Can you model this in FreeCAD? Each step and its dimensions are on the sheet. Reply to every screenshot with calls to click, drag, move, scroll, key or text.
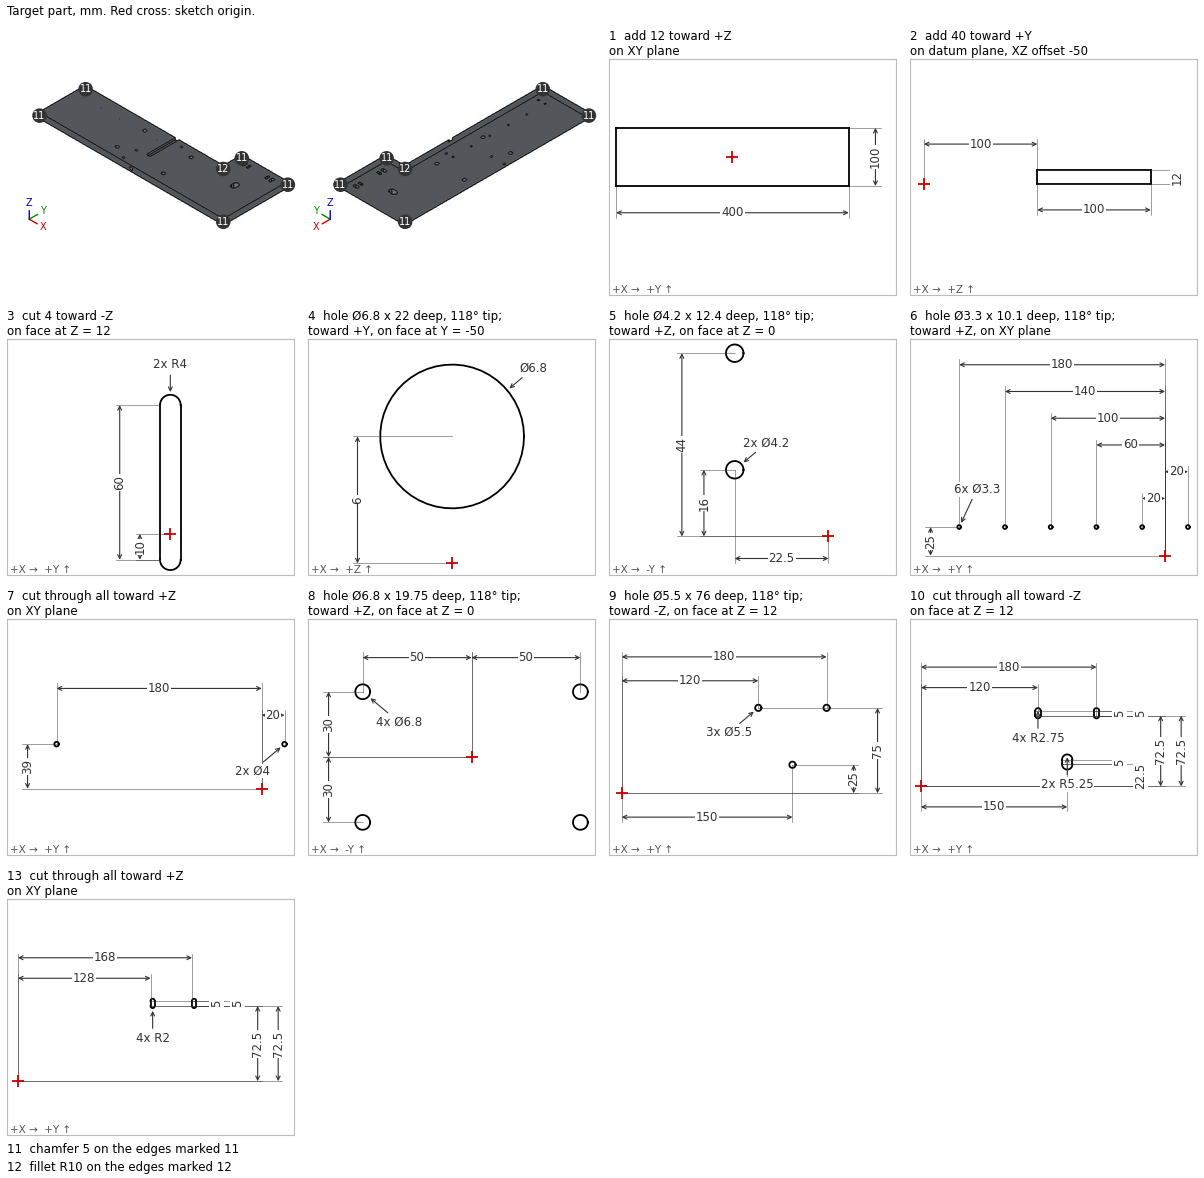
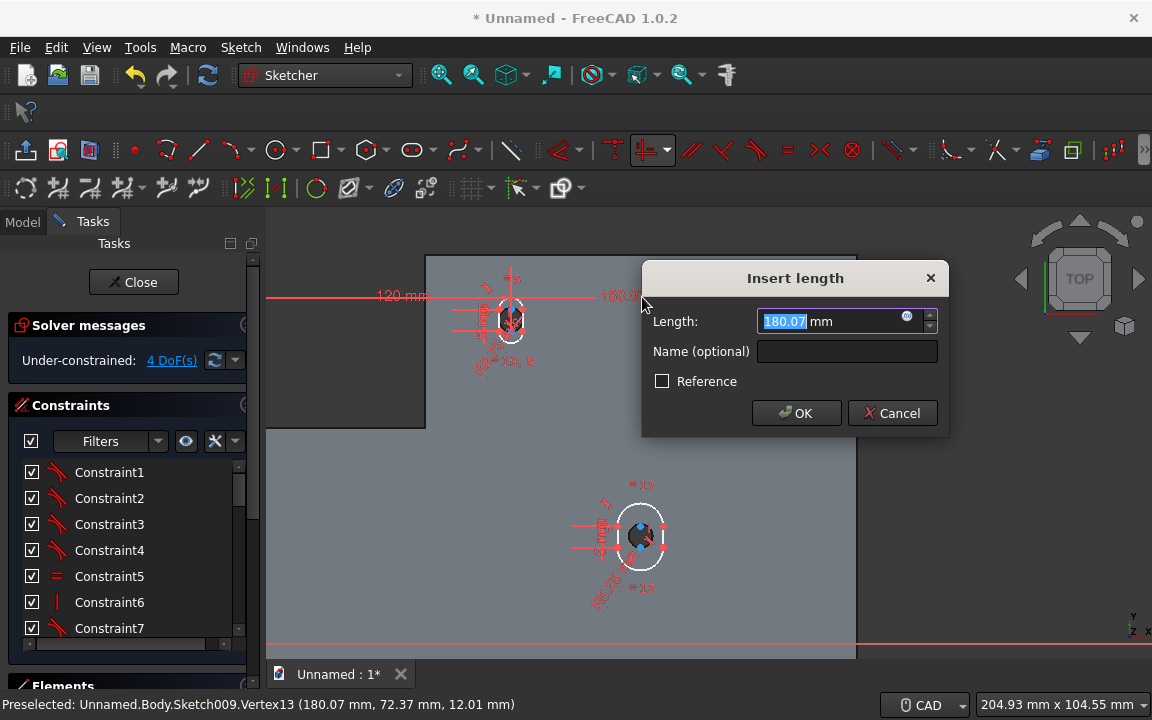
text(180)
key(Return)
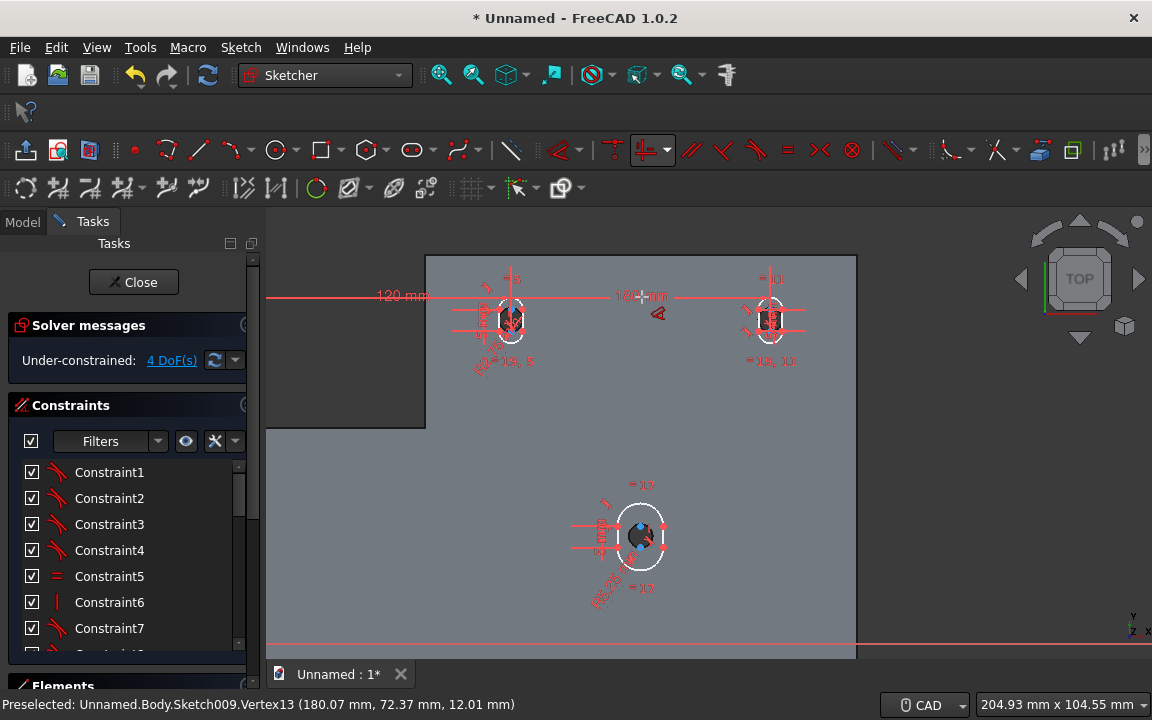
click(640, 548)
click(467, 514)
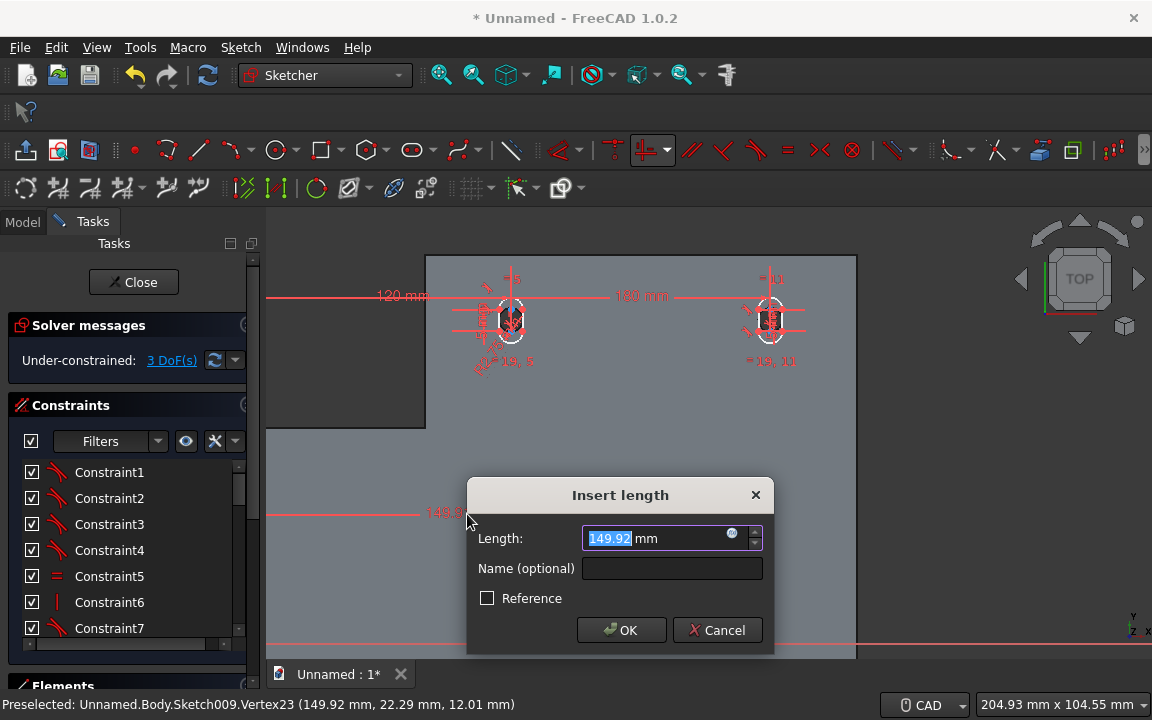
text(150)
key(Return)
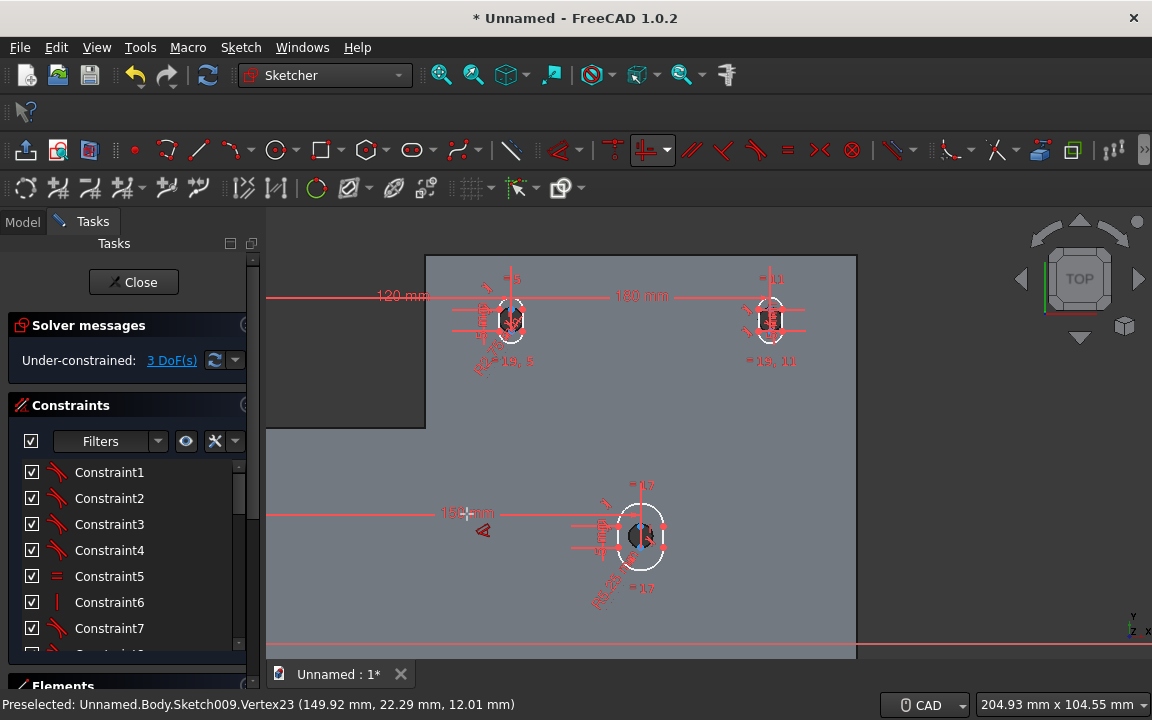
click(499, 331)
click(533, 481)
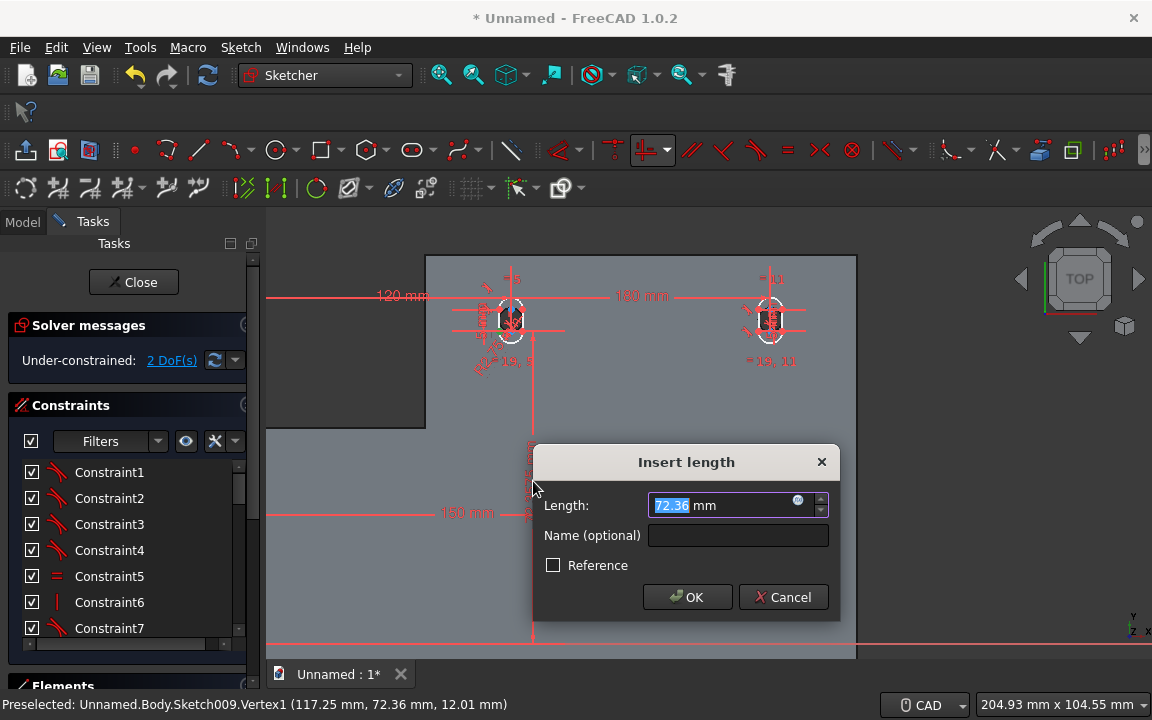
text(72.5)
key(Return)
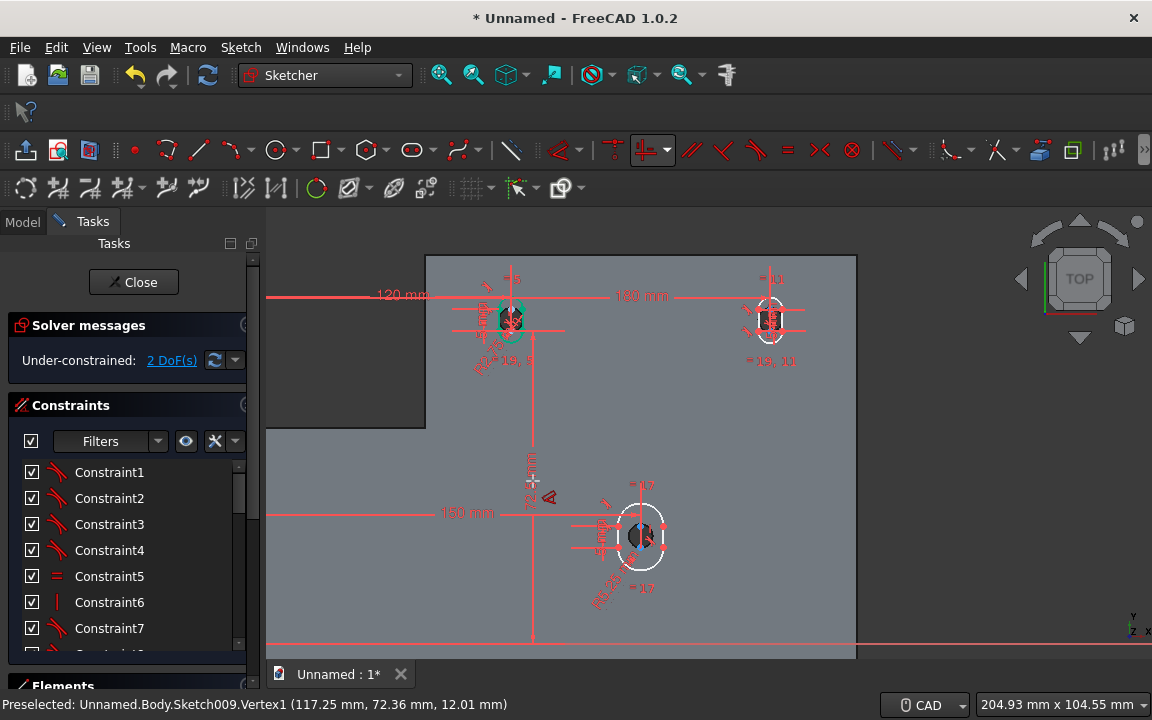
click(759, 331)
click(793, 481)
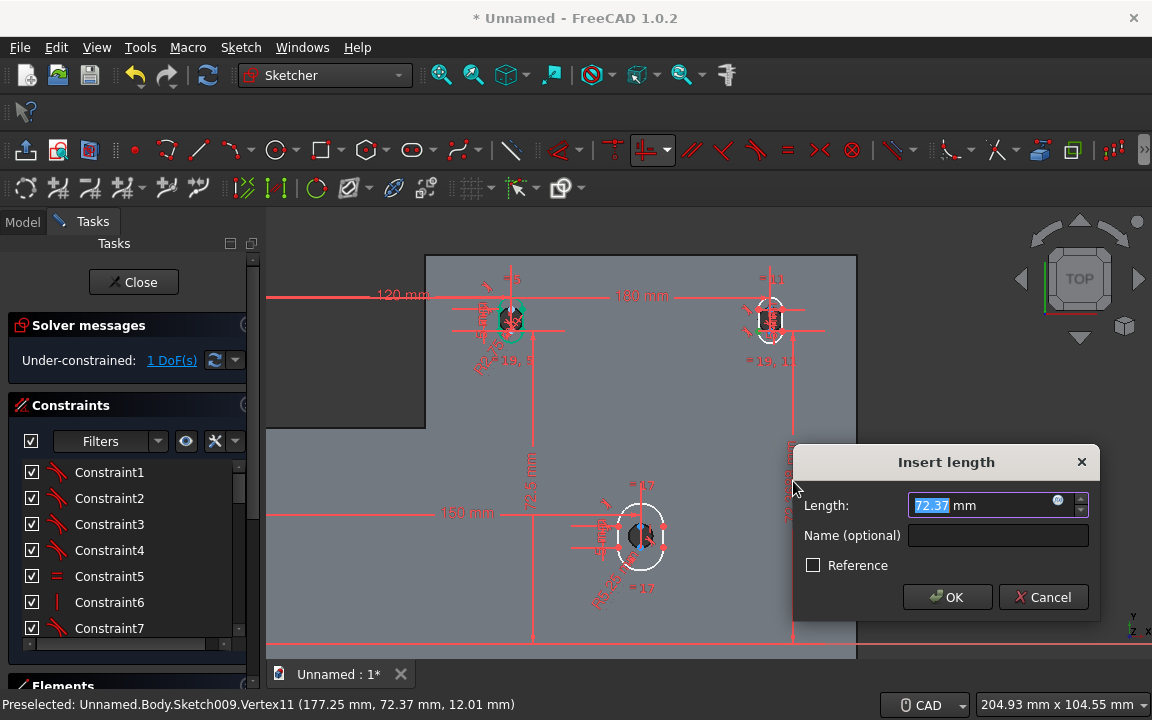
text(72.5)
key(Return)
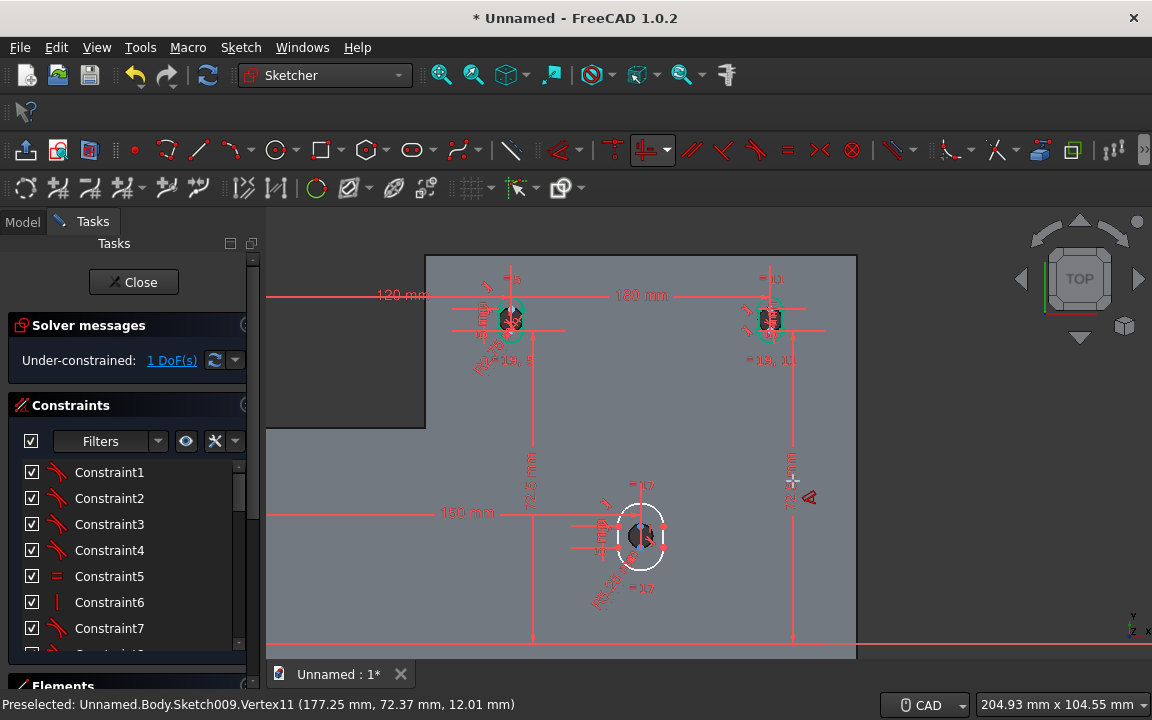
click(618, 548)
click(652, 609)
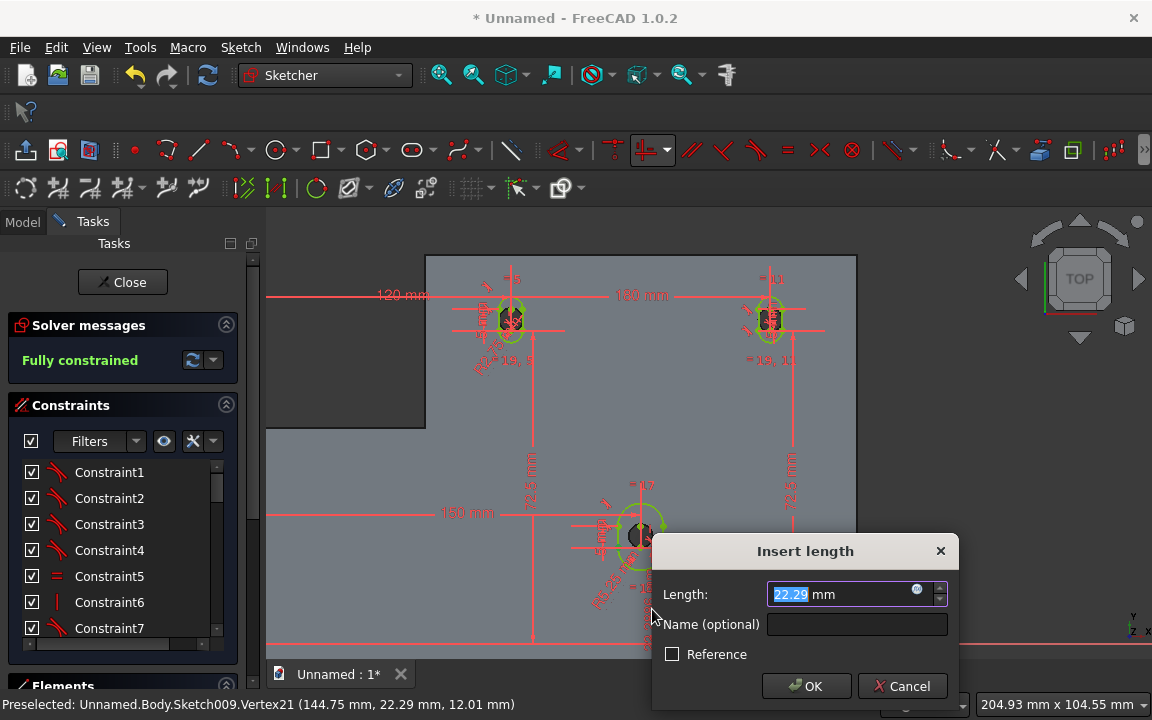
text(22.5)
key(Return)
key(Escape)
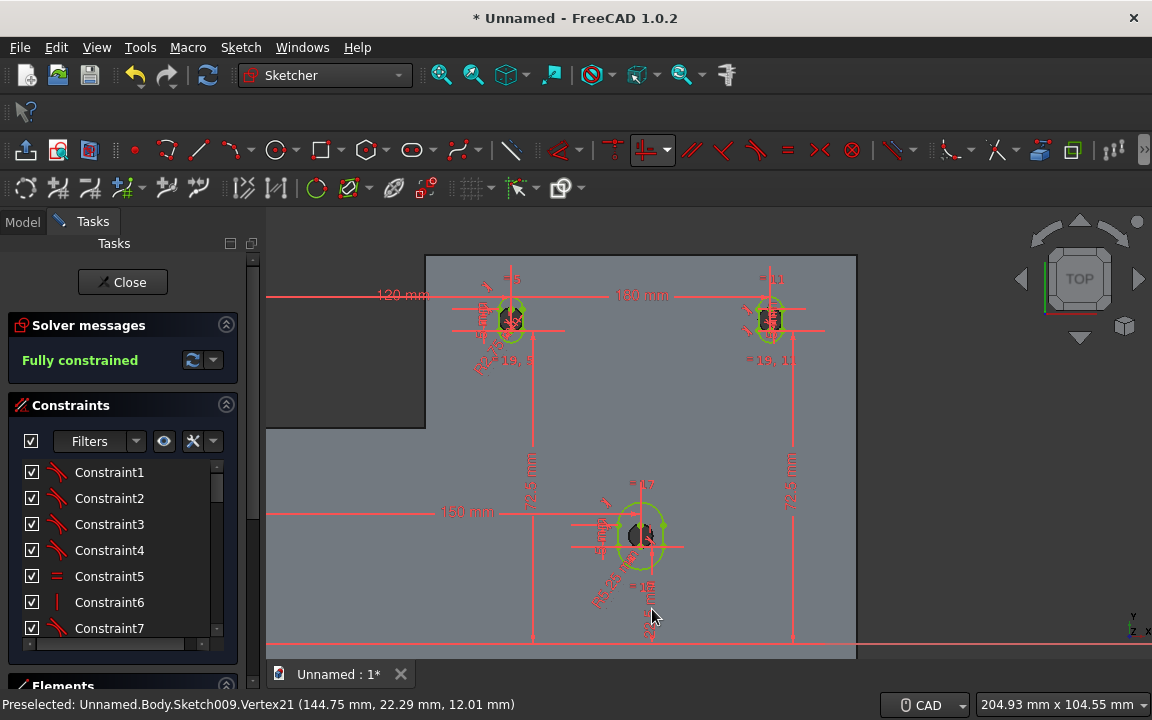
click(123, 282)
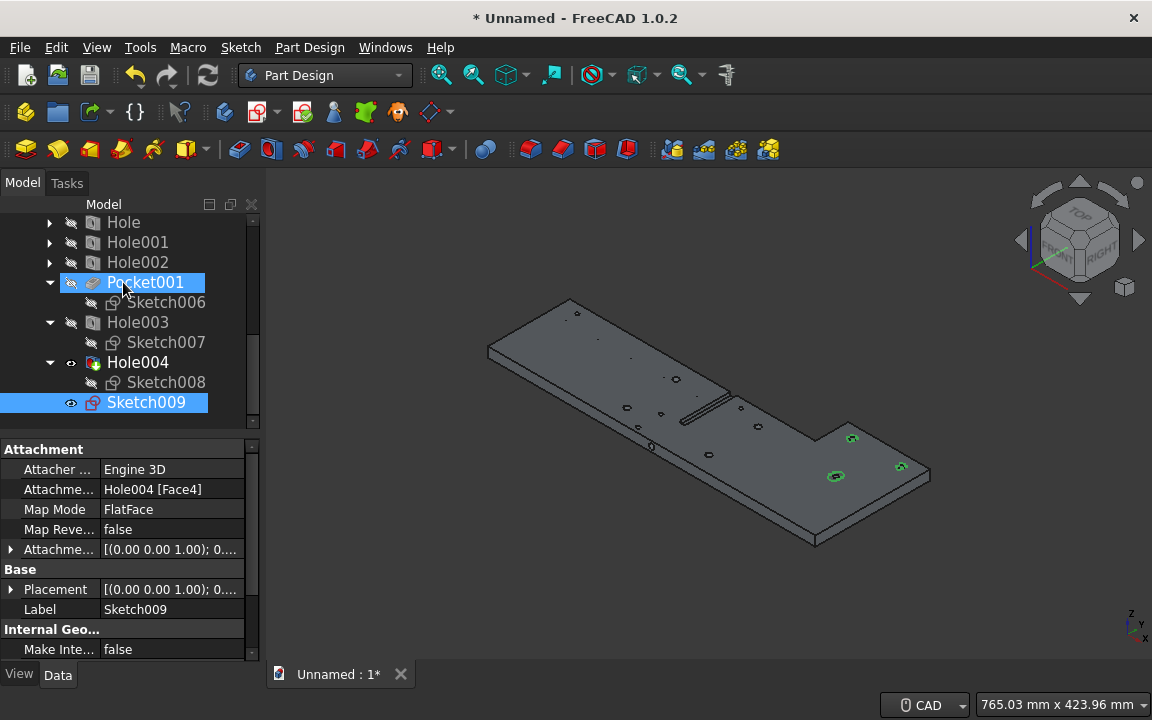
click(240, 150)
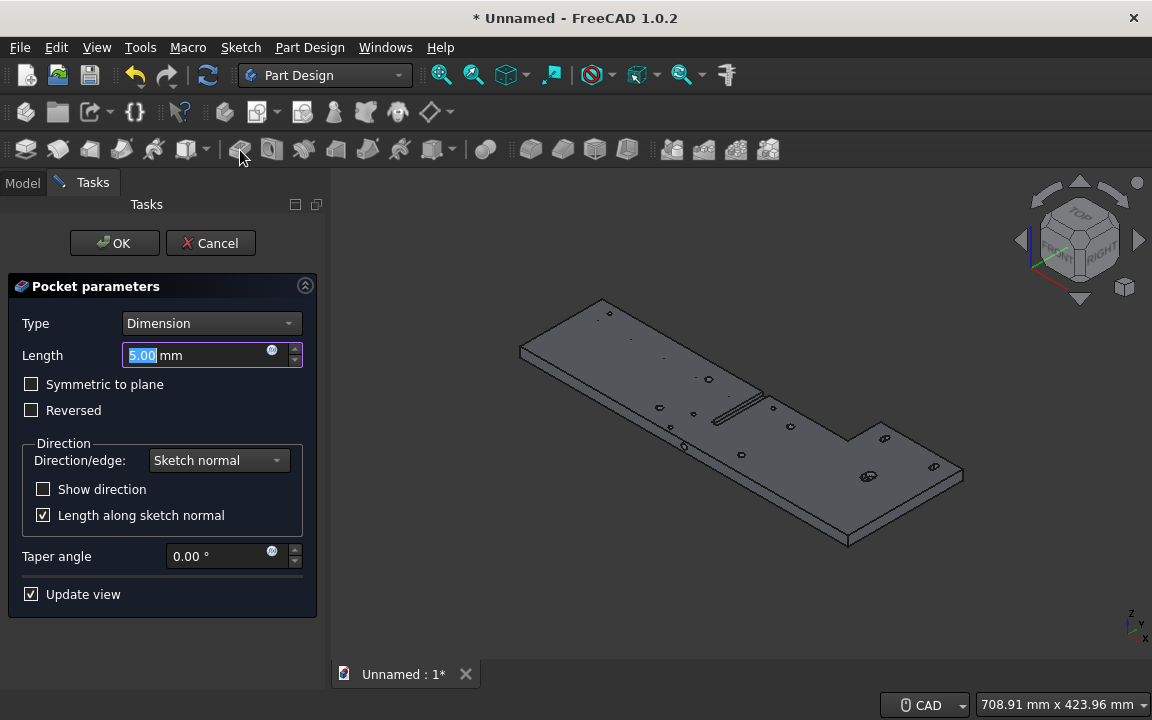
click(212, 324)